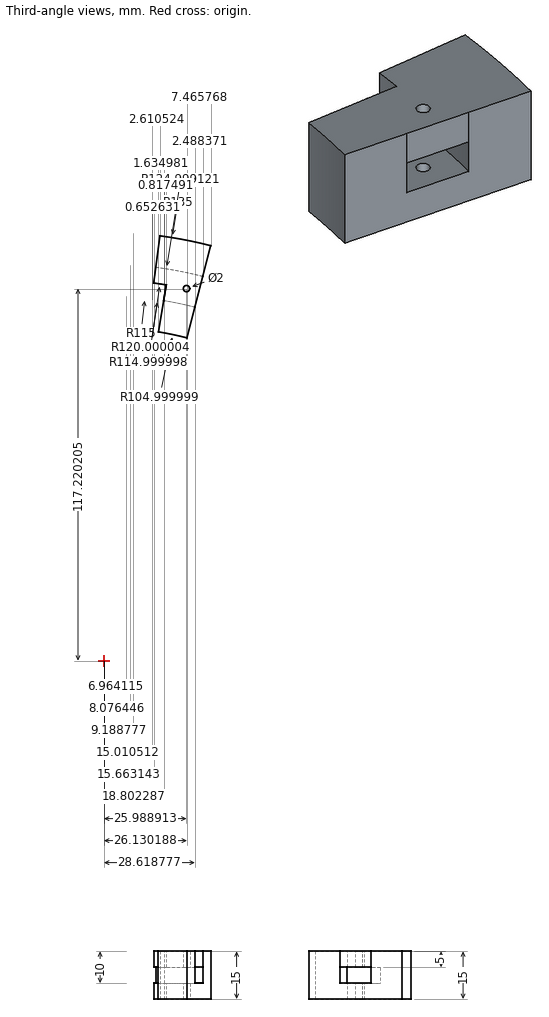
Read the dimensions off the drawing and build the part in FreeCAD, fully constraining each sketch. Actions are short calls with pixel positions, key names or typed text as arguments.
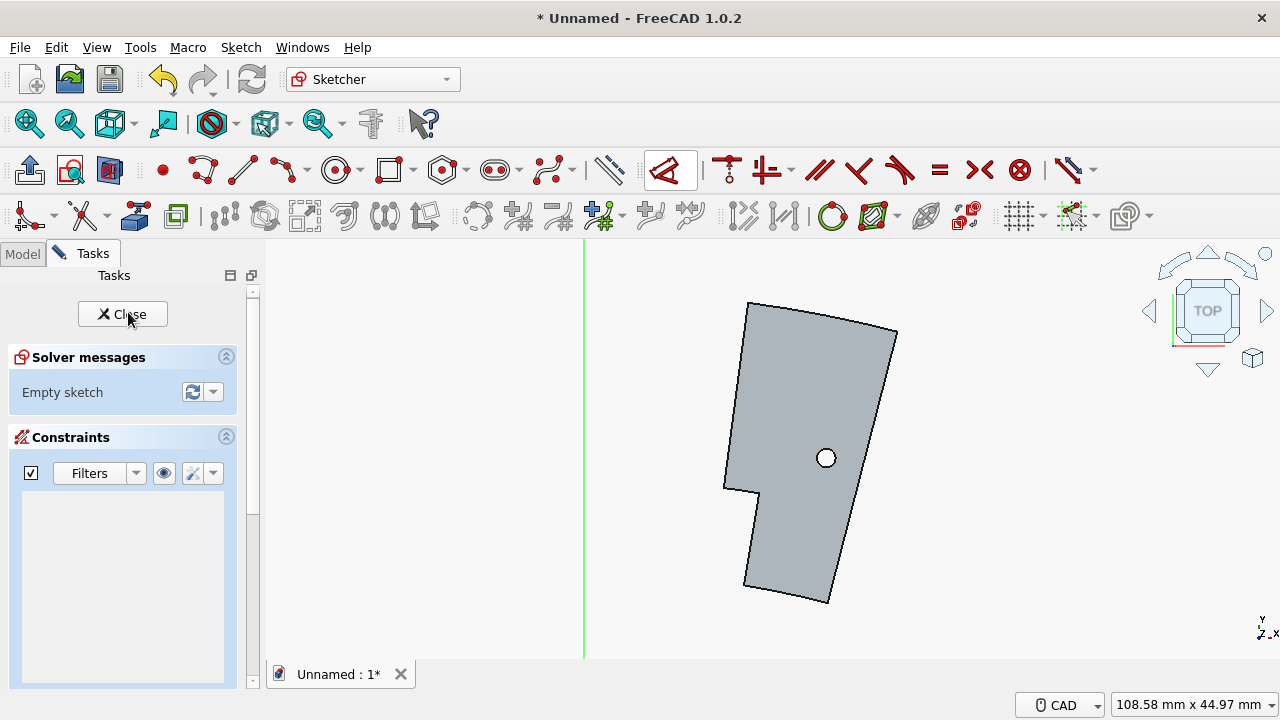
key(q)
key(s)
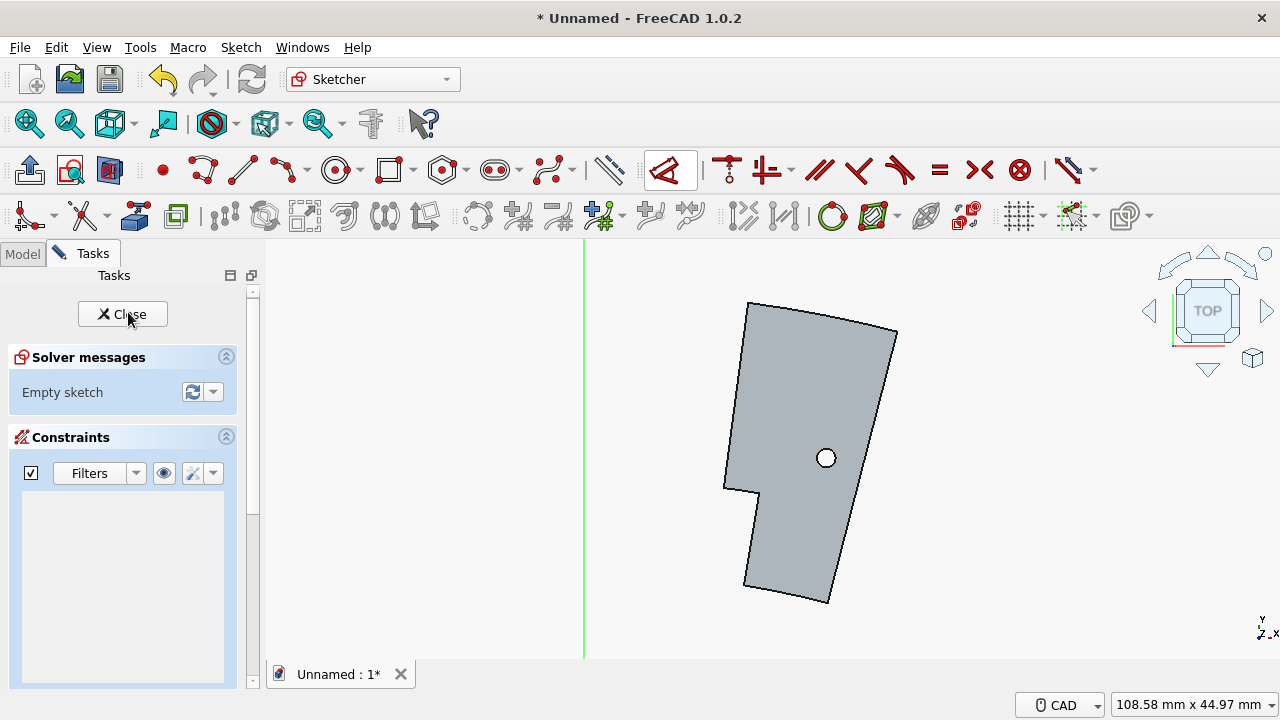
scroll(756, 472, up, 8)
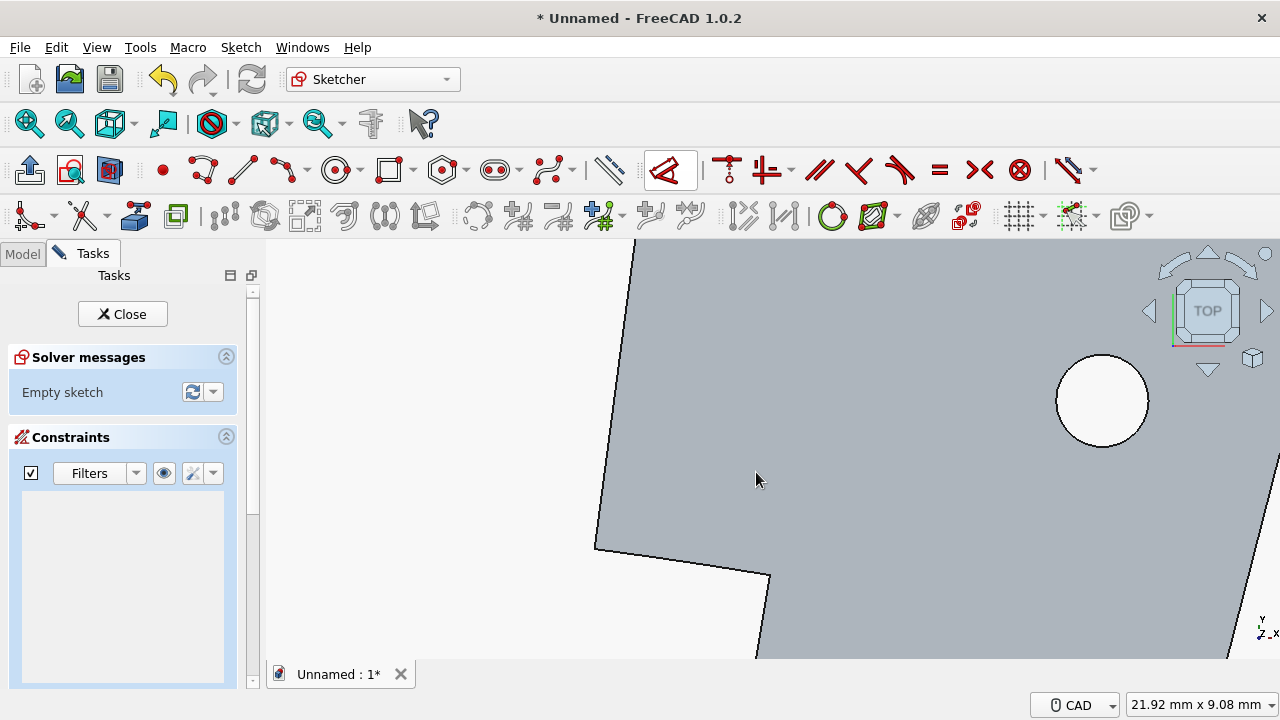
key(g)
key(l)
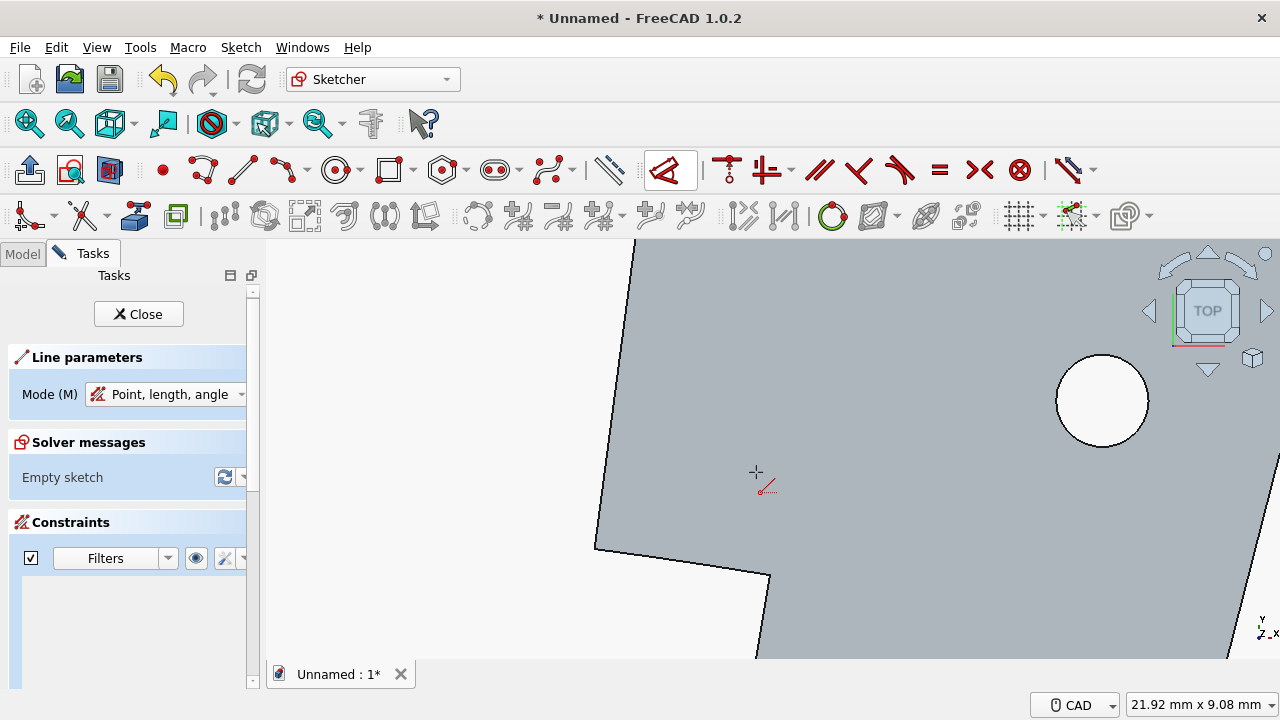
click(625, 320)
click(595, 549)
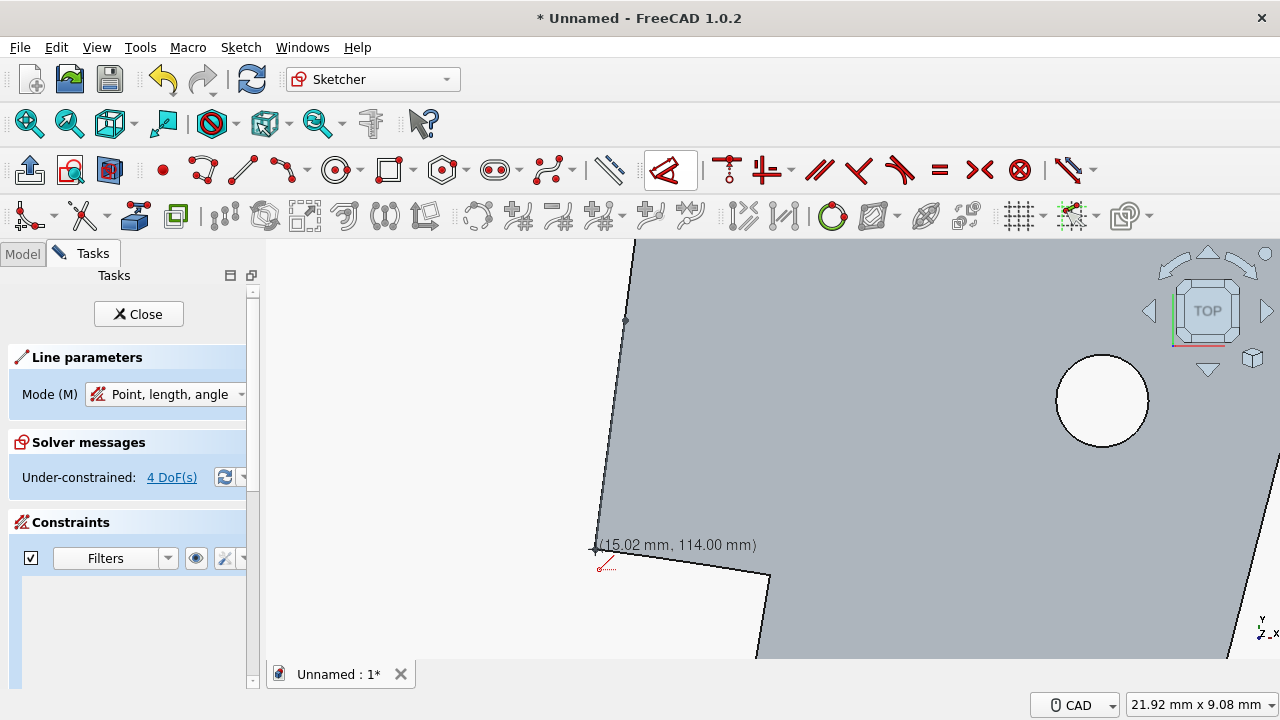
click(770, 575)
click(808, 347)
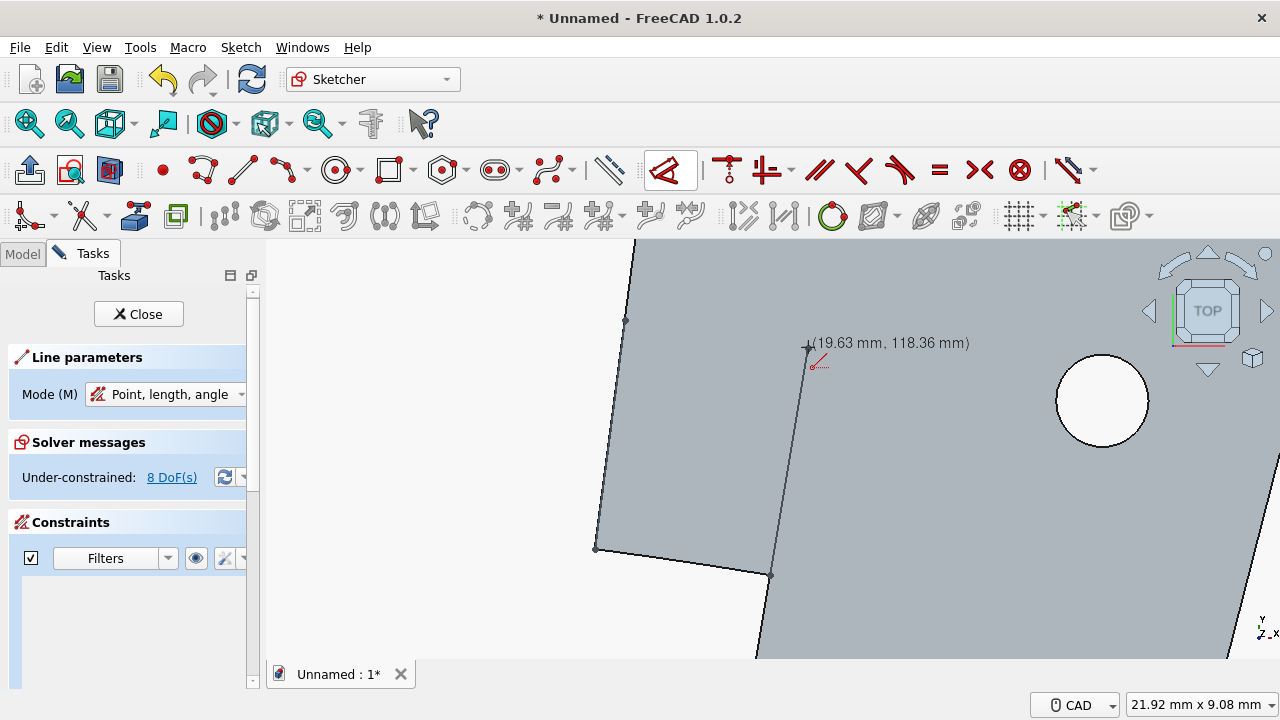
click(284, 170)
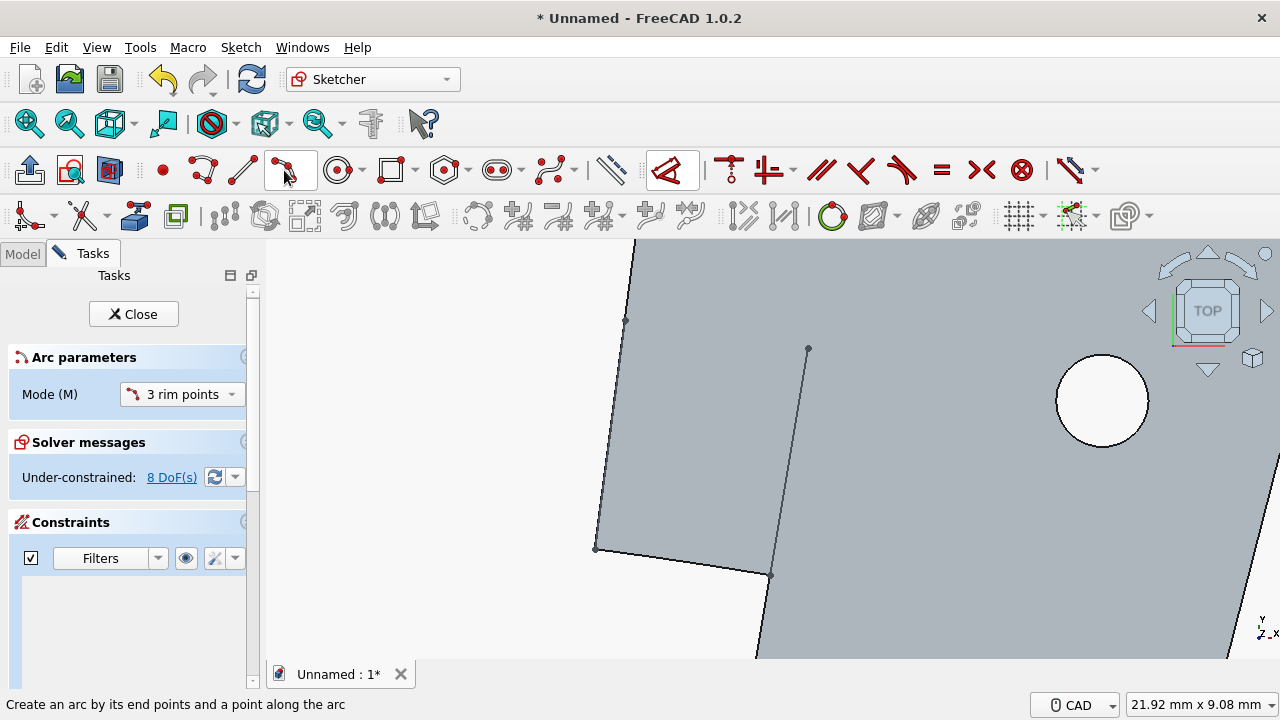
click(595, 550)
click(770, 576)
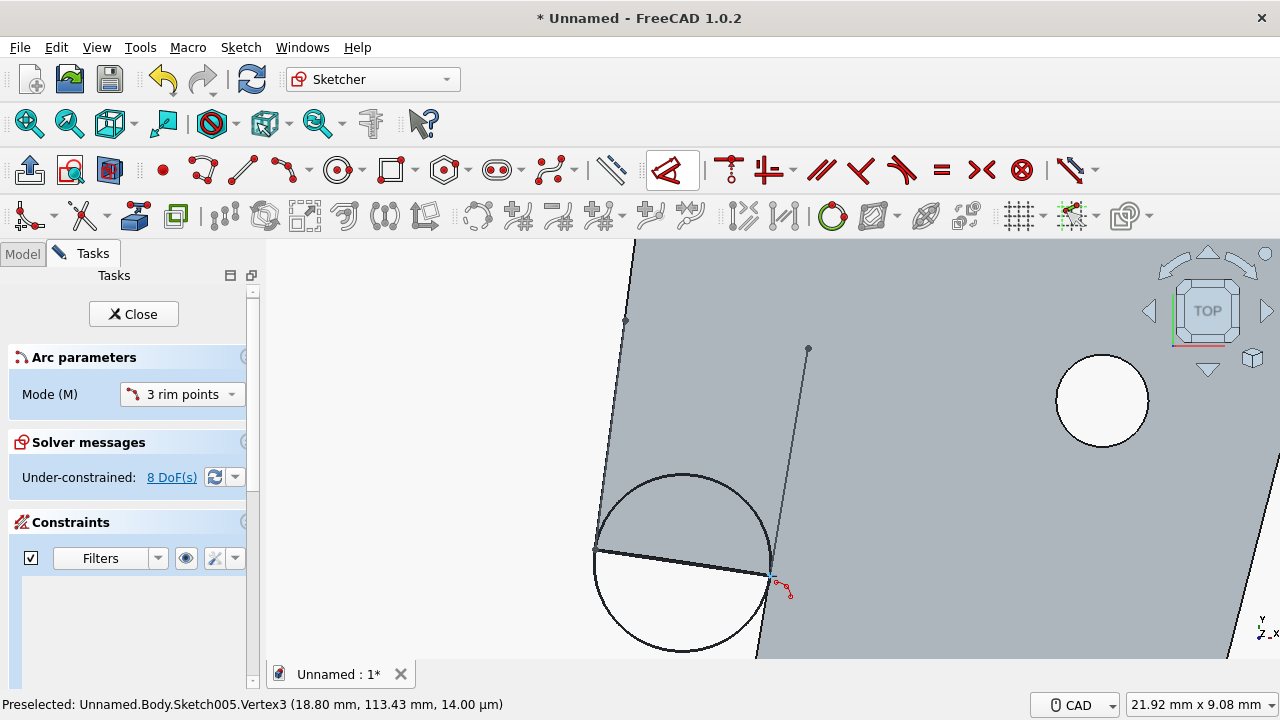
scroll(682, 561, up, 16)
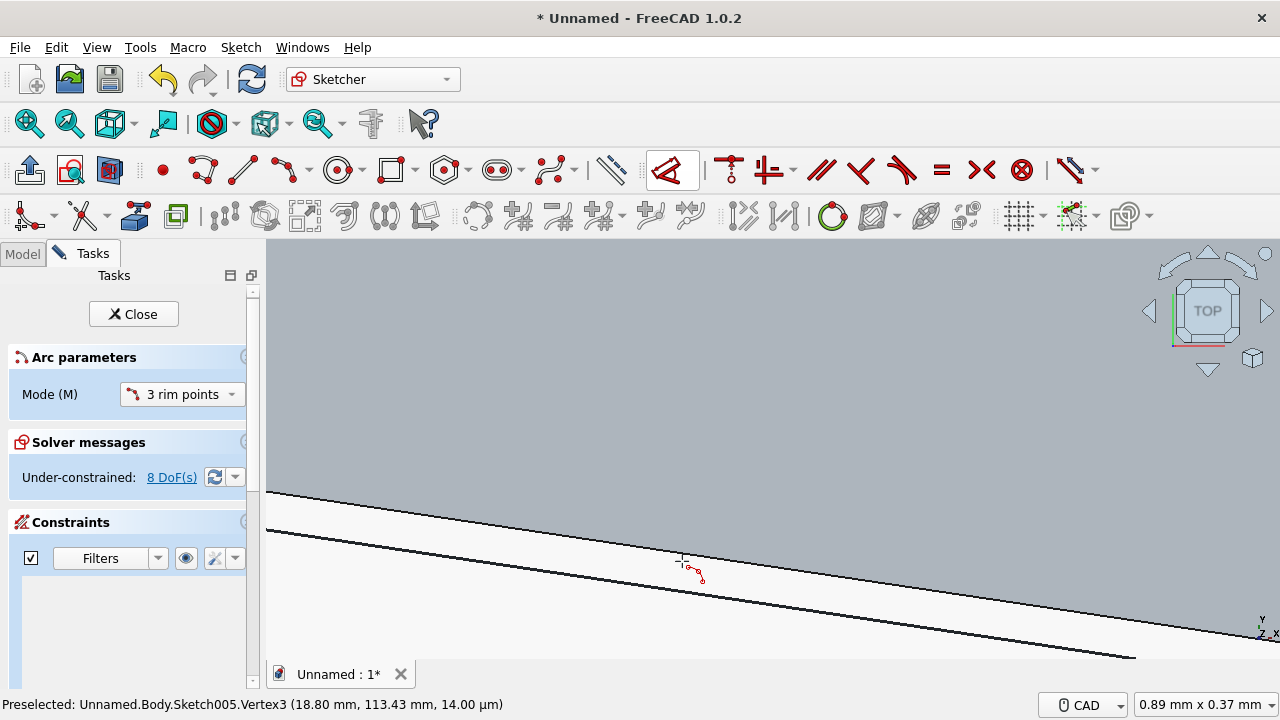
click(681, 551)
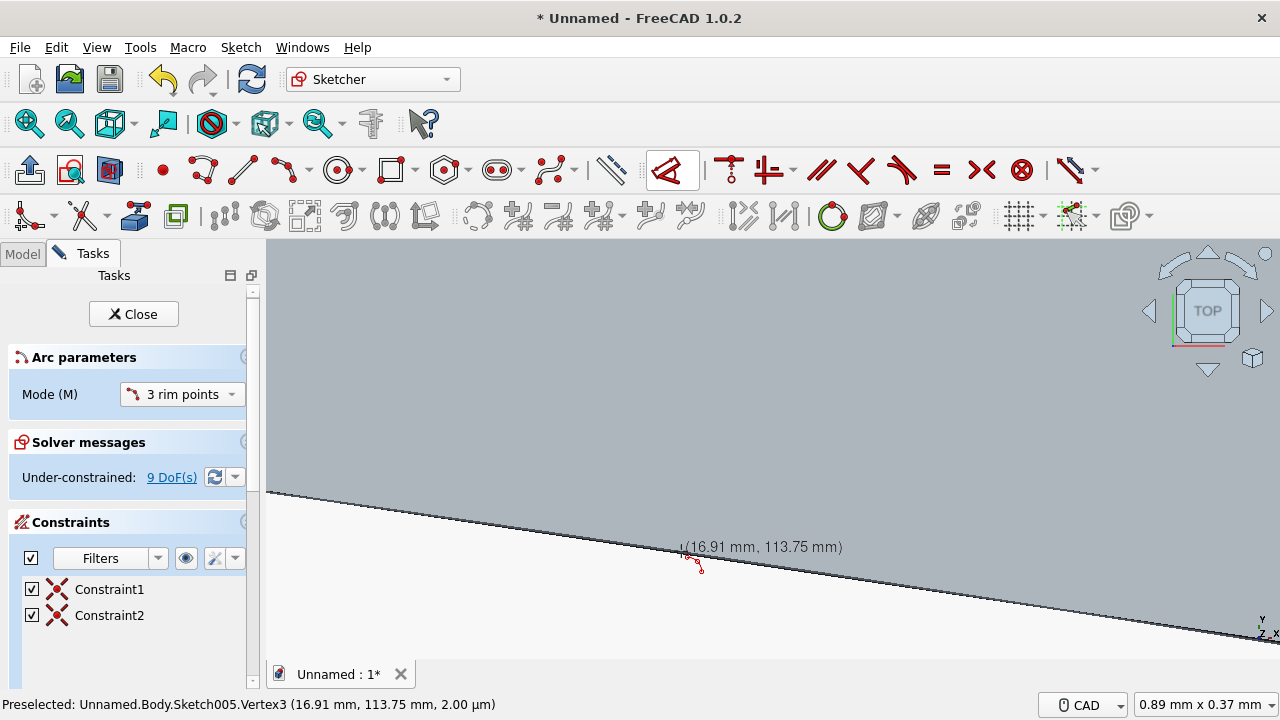
scroll(682, 590, down, 15)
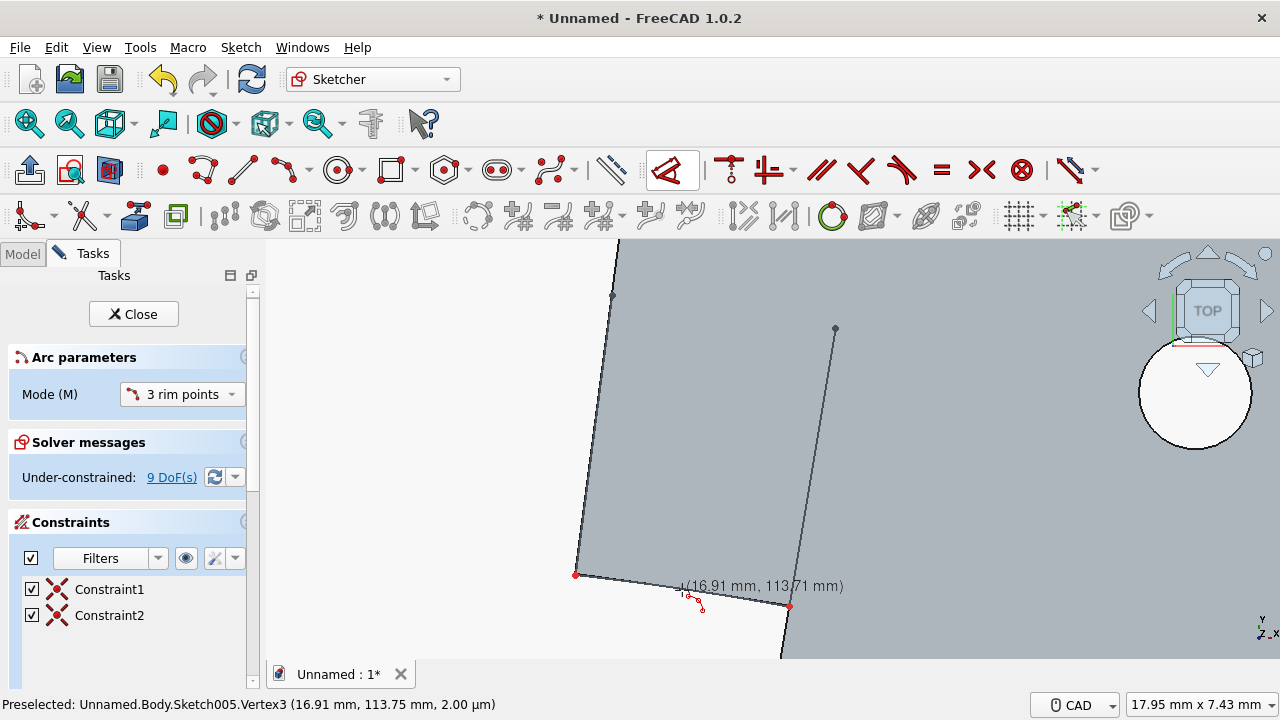
click(836, 328)
click(612, 295)